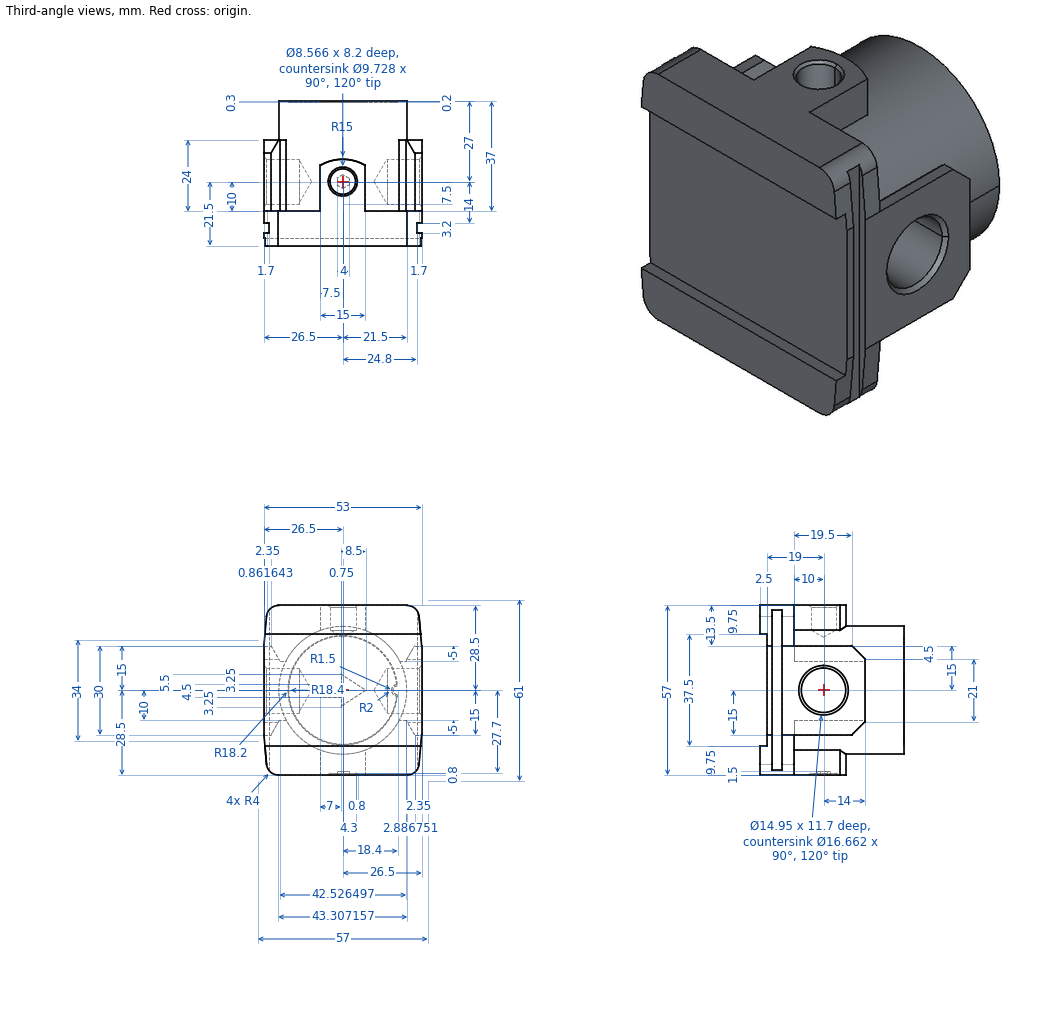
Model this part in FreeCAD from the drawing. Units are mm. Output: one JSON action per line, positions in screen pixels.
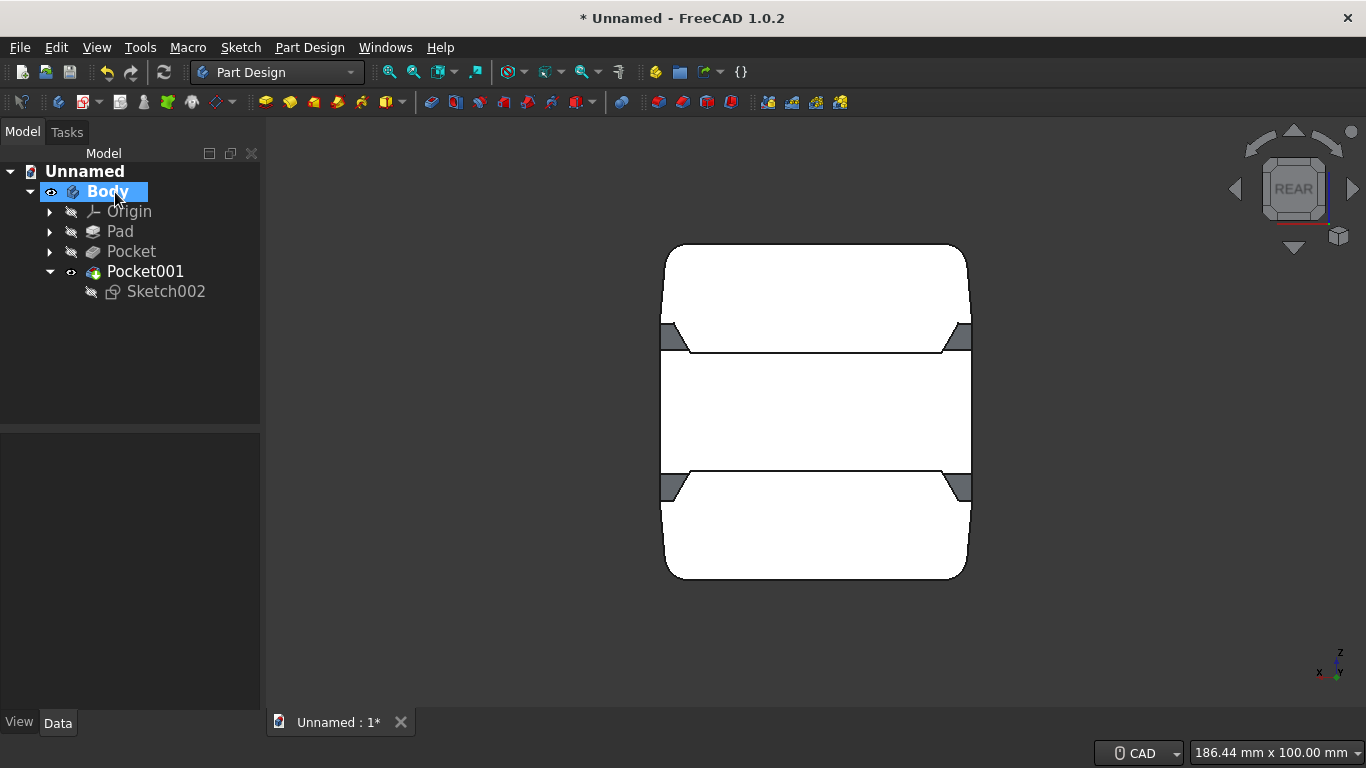
{"action": "left_click", "coordinate": [84, 102]}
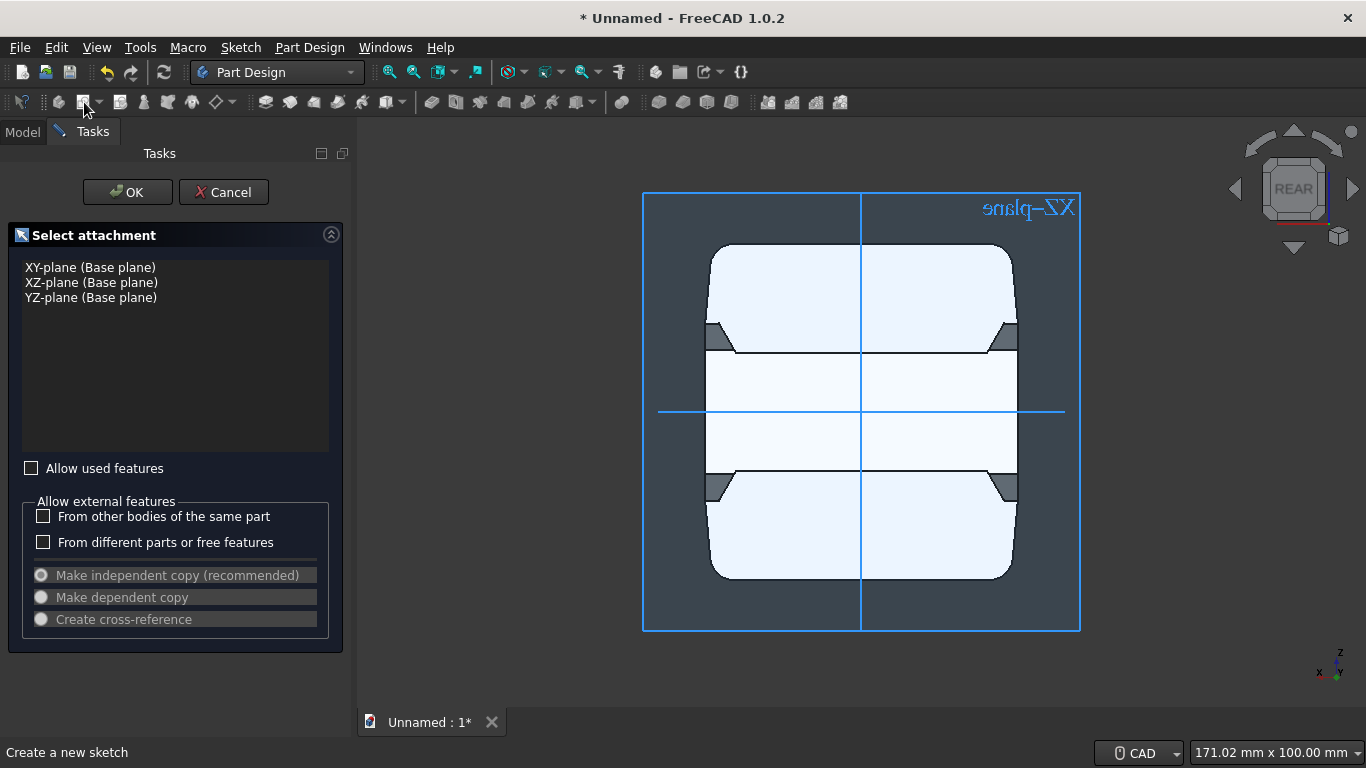
{"action": "left_click", "coordinate": [82, 268]}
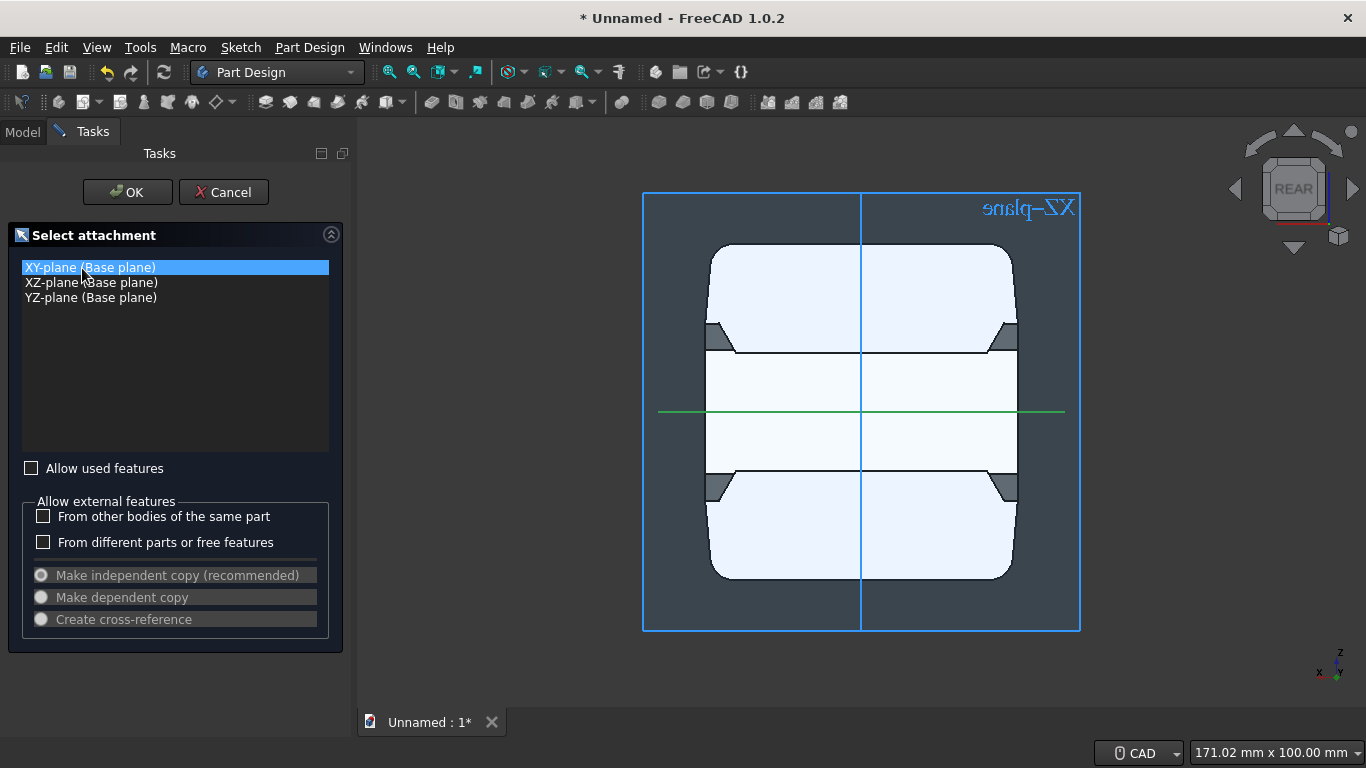
{"action": "left_click", "coordinate": [128, 192]}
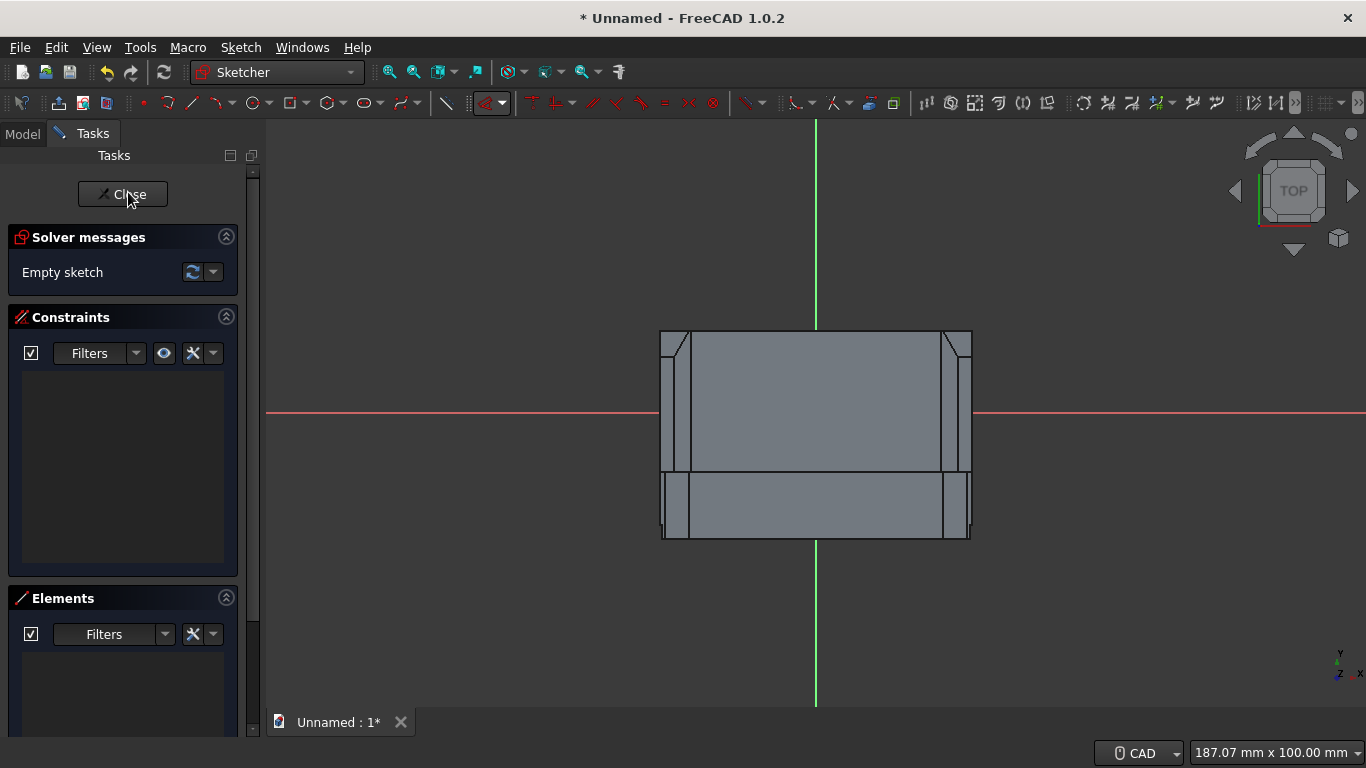
{"action": "left_click", "coordinate": [108, 104]}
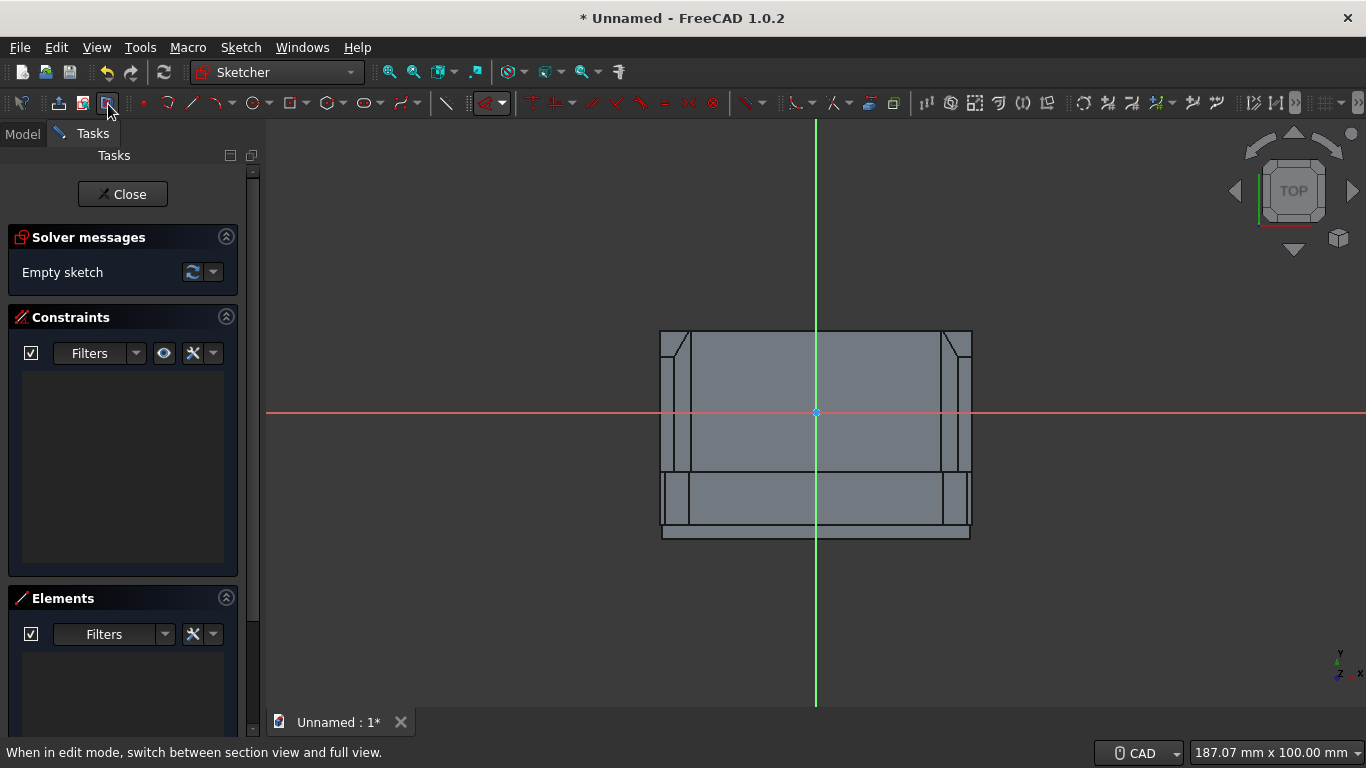
{"action": "scroll", "coordinate": [846, 424], "scroll_direction": "up", "scroll_amount": 6}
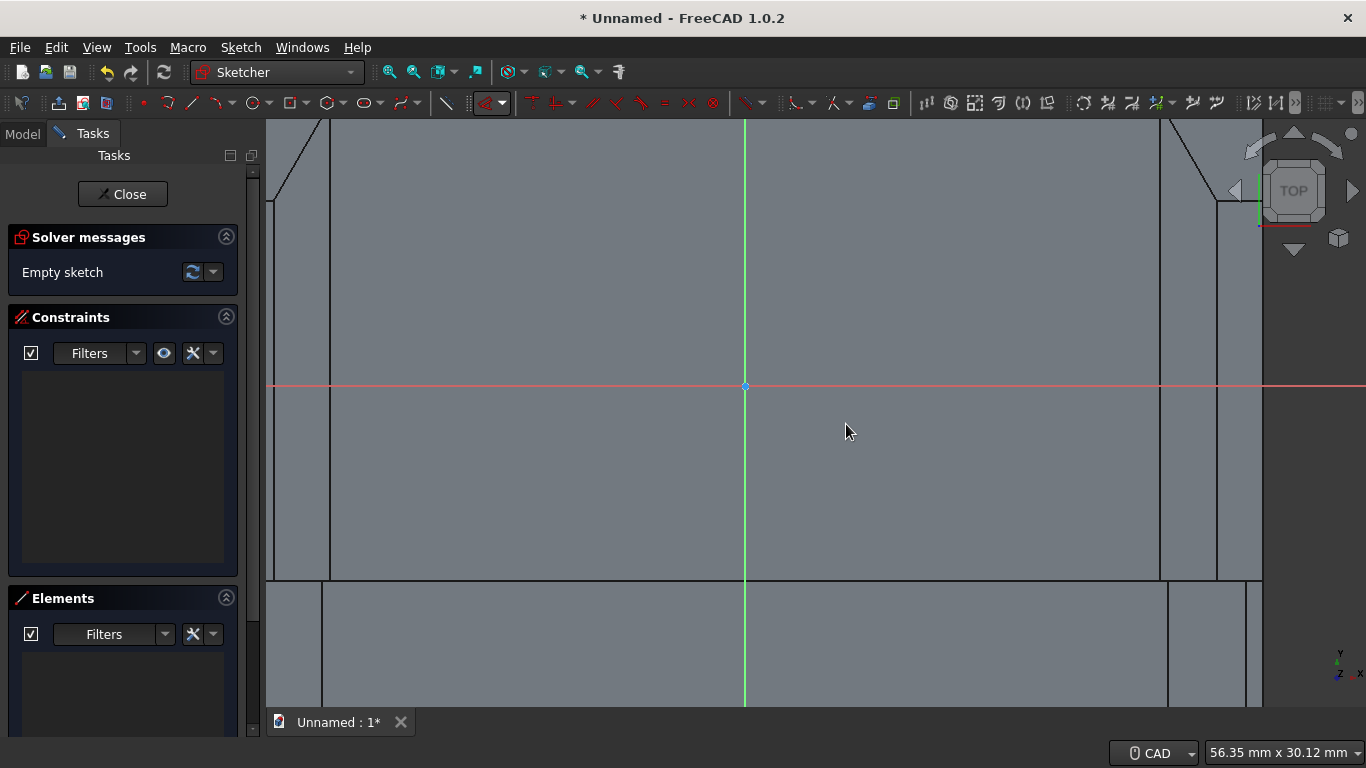
{"action": "left_click", "coordinate": [168, 104]}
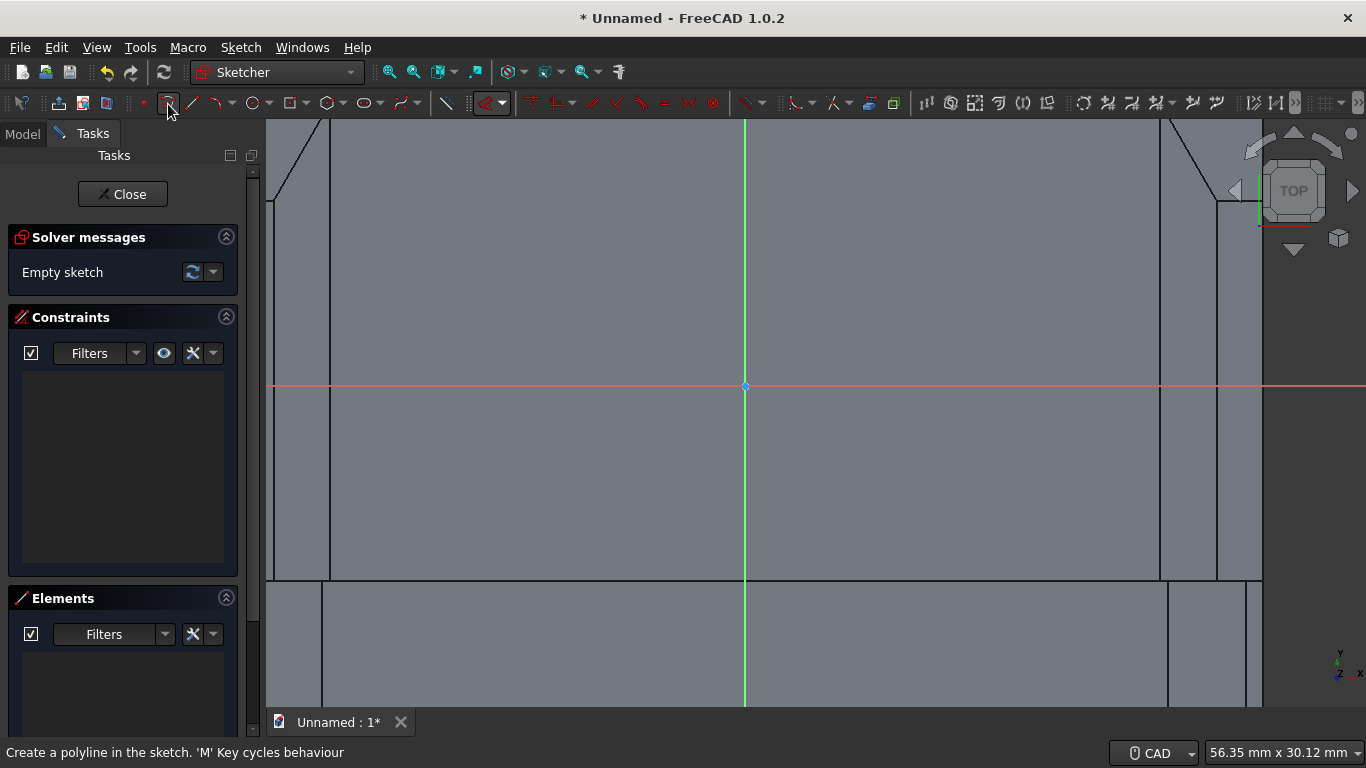
{"action": "left_click", "coordinate": [599, 279]}
{"action": "left_click", "coordinate": [599, 581]}
{"action": "left_click", "coordinate": [892, 581]}
{"action": "left_click", "coordinate": [892, 279]}
{"action": "right_click", "coordinate": [892, 279]}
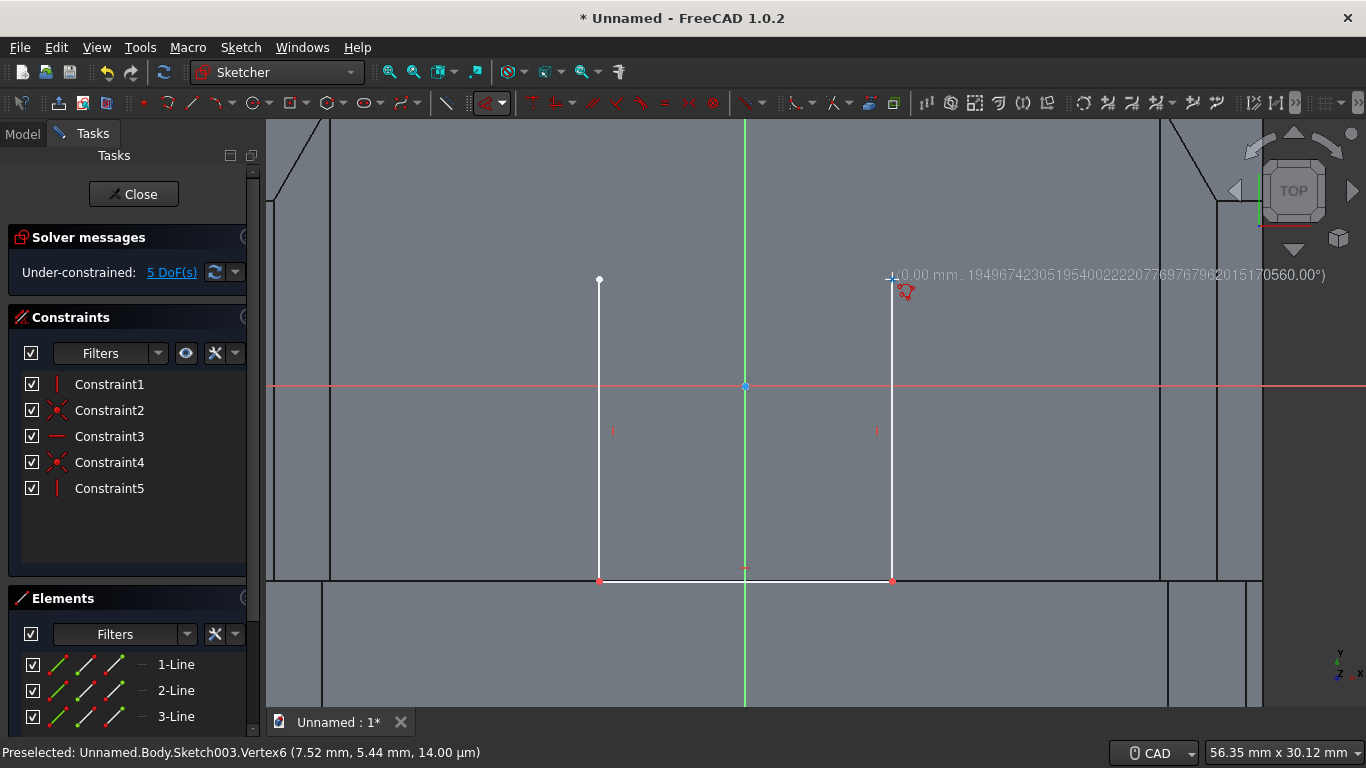
{"action": "key", "text": "g 3 a"}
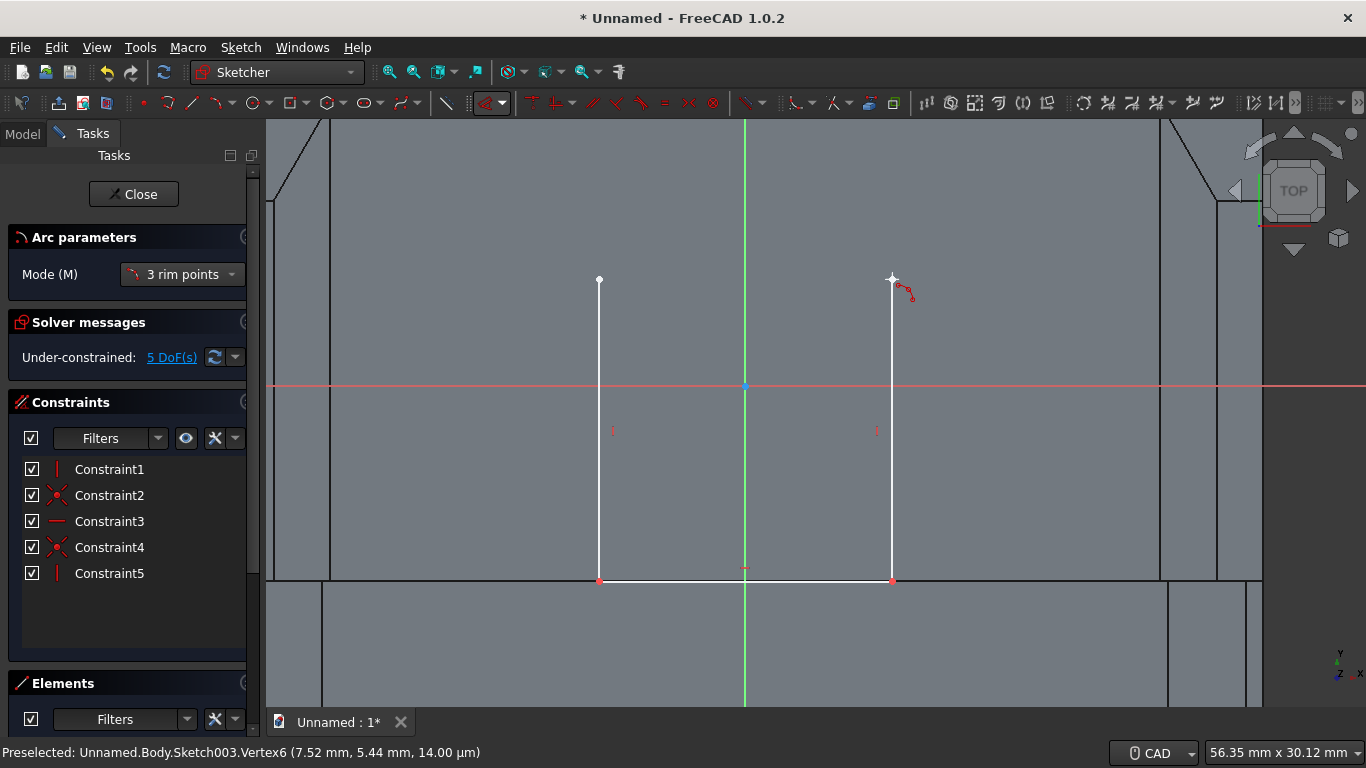
{"action": "left_click", "coordinate": [892, 280]}
{"action": "left_click", "coordinate": [599, 280]}
{"action": "left_click", "coordinate": [776, 241]}
{"action": "key", "text": "Escape"}